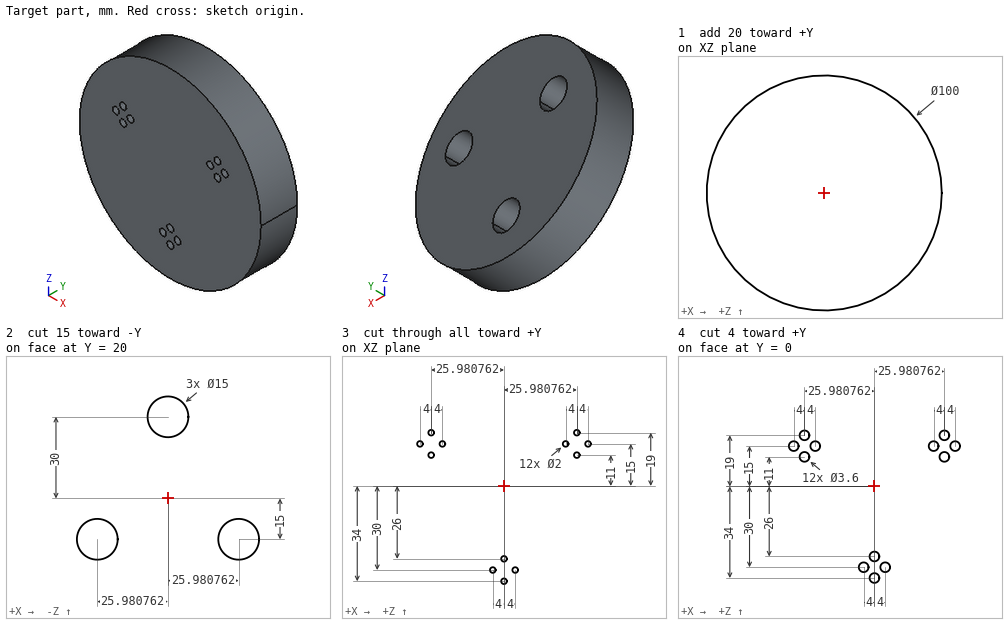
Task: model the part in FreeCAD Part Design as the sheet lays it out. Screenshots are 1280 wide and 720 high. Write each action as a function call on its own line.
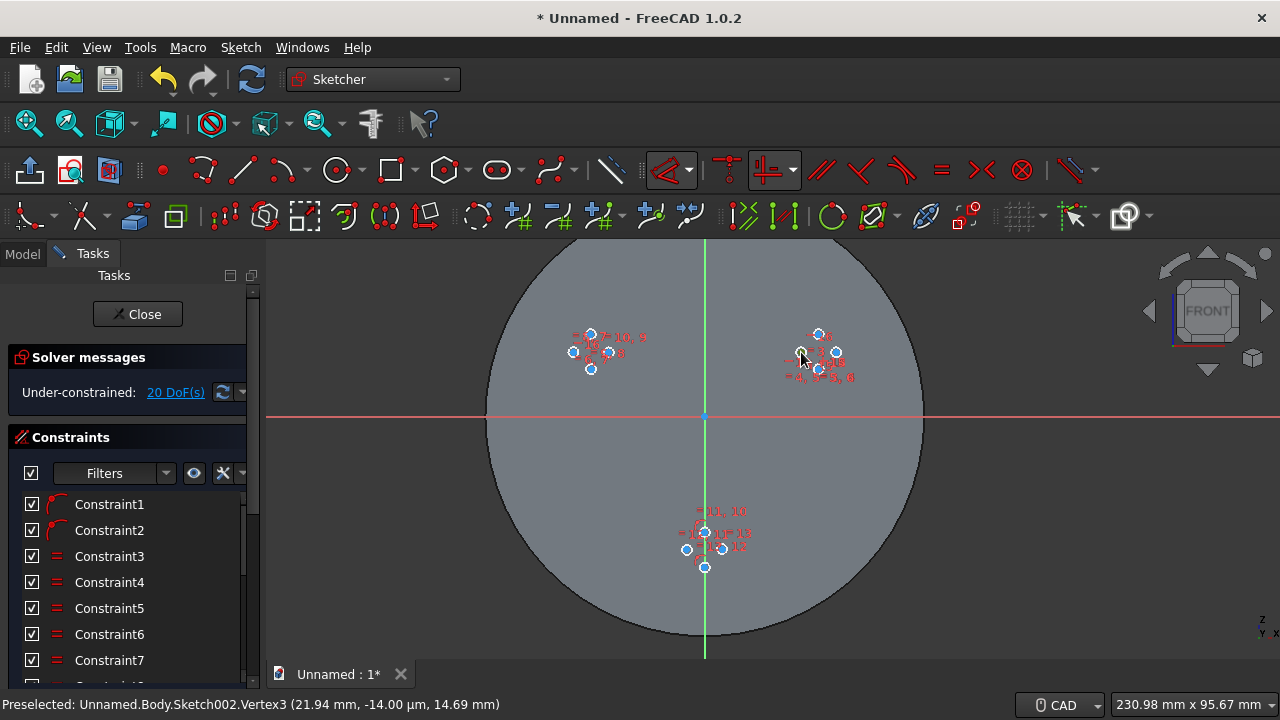
click(571, 354)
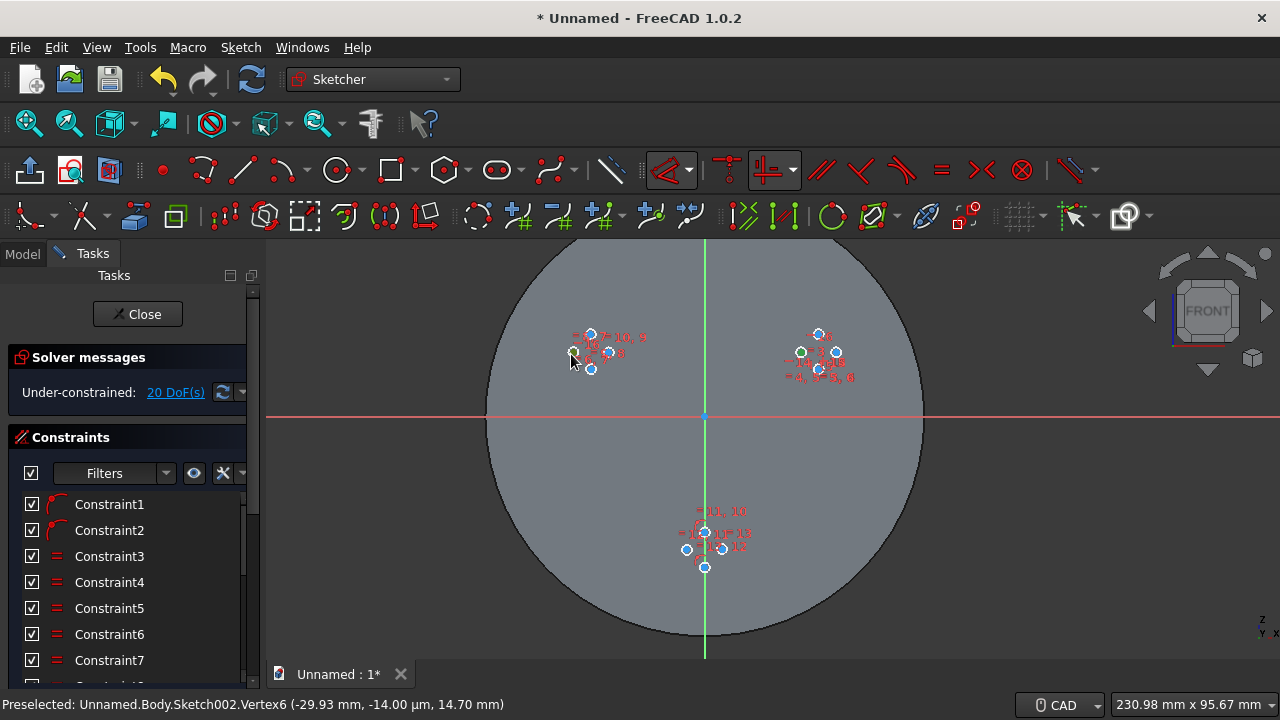
key(h)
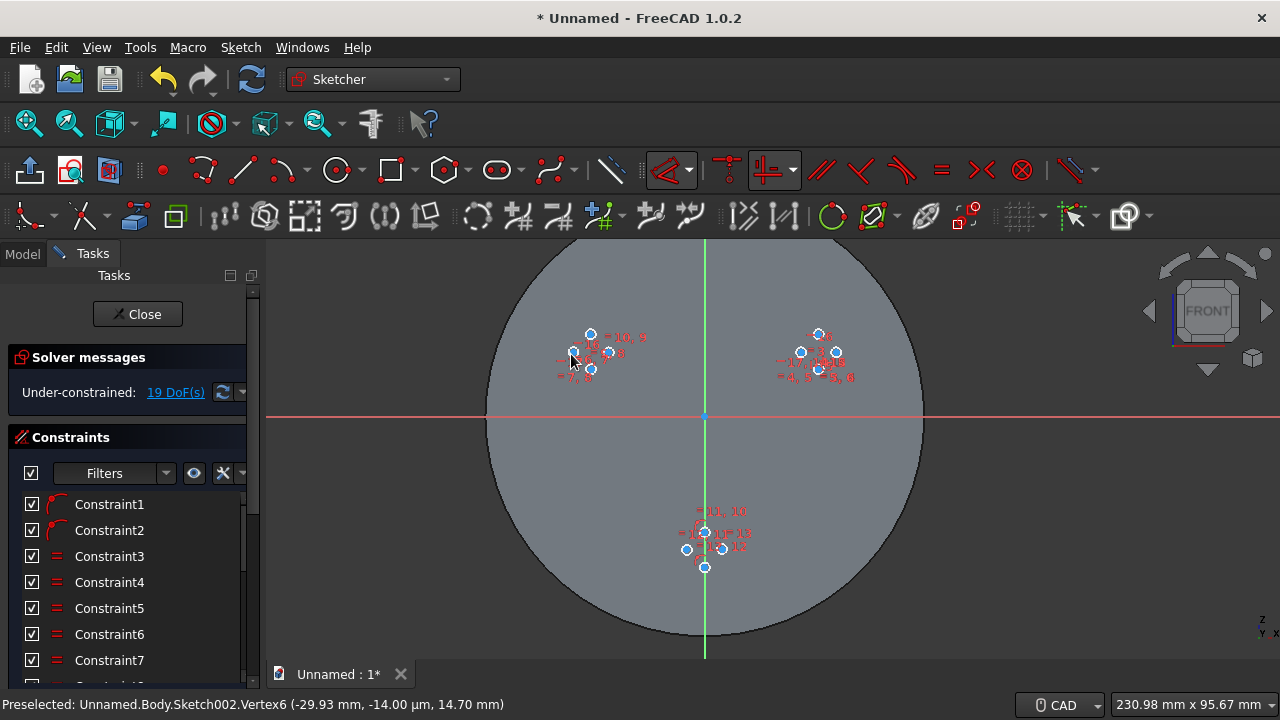
click(591, 334)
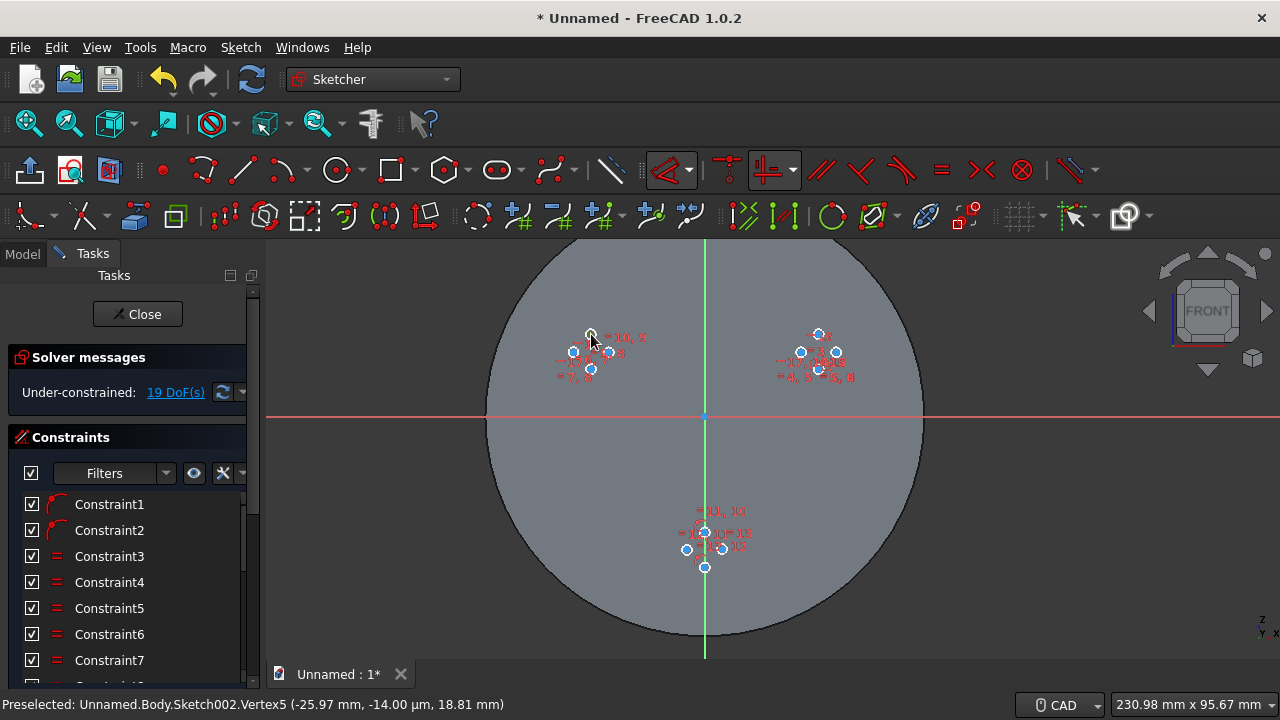
click(593, 371)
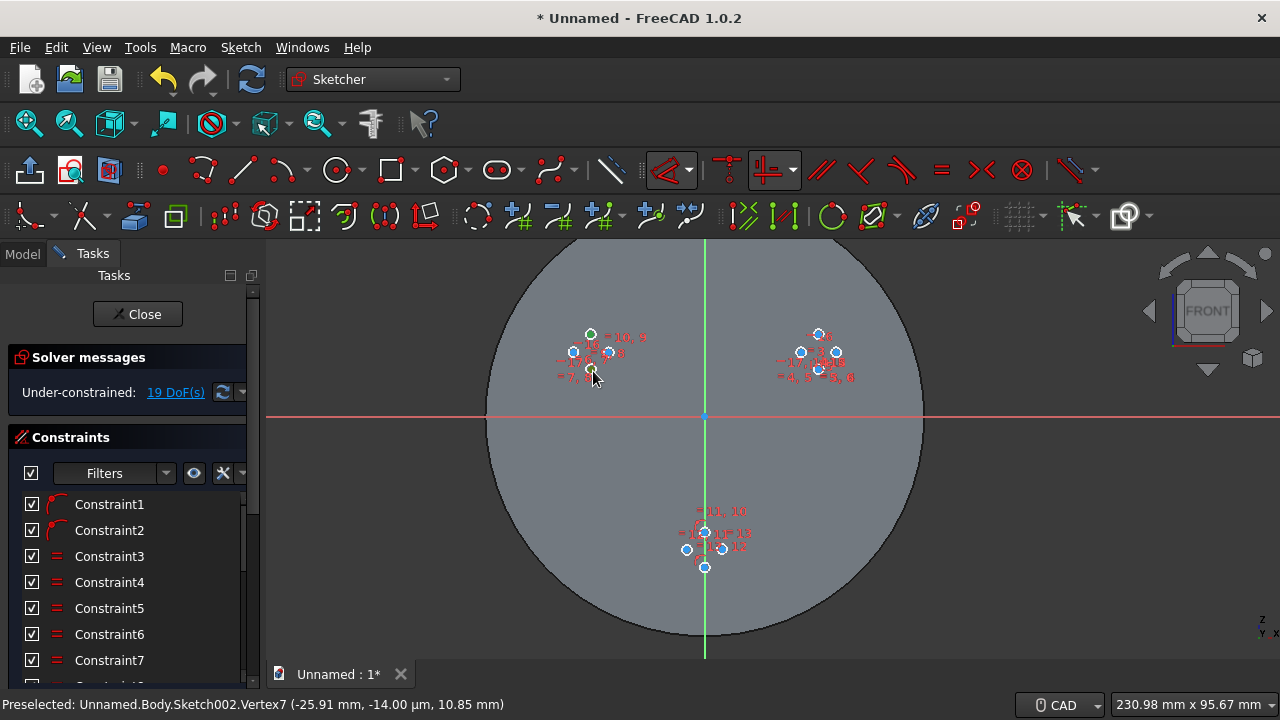
click(796, 170)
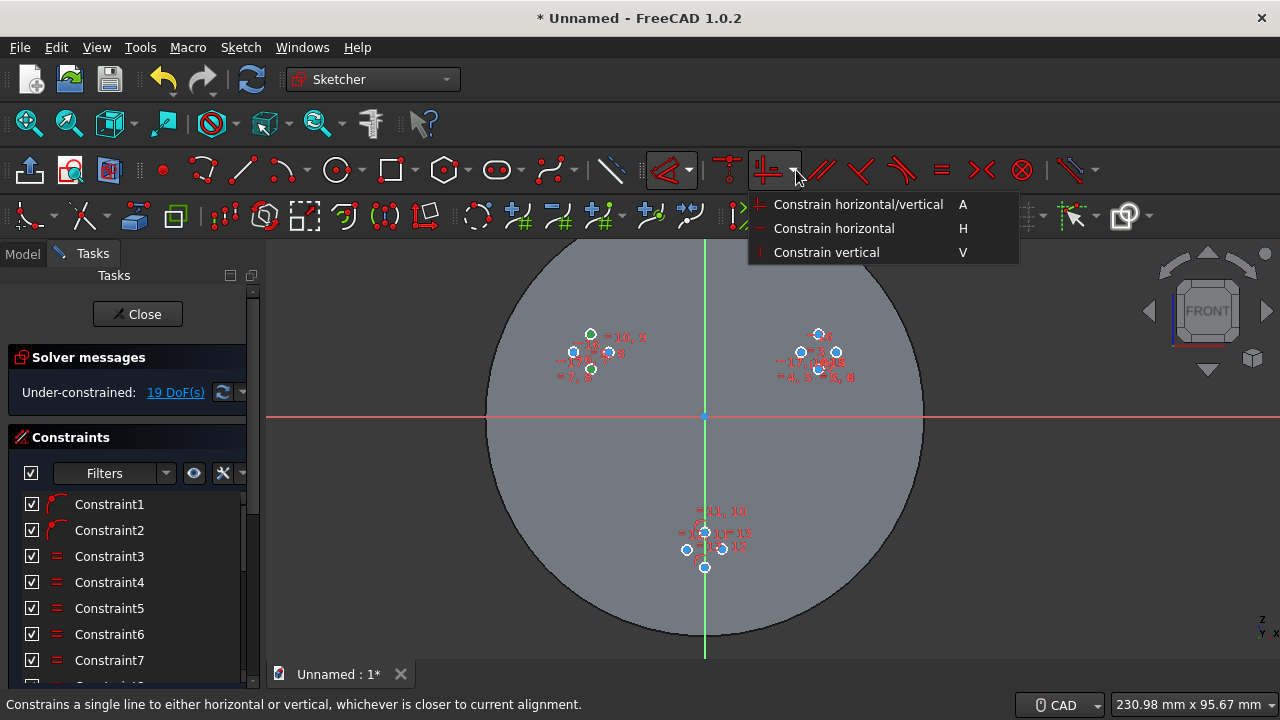
click(884, 252)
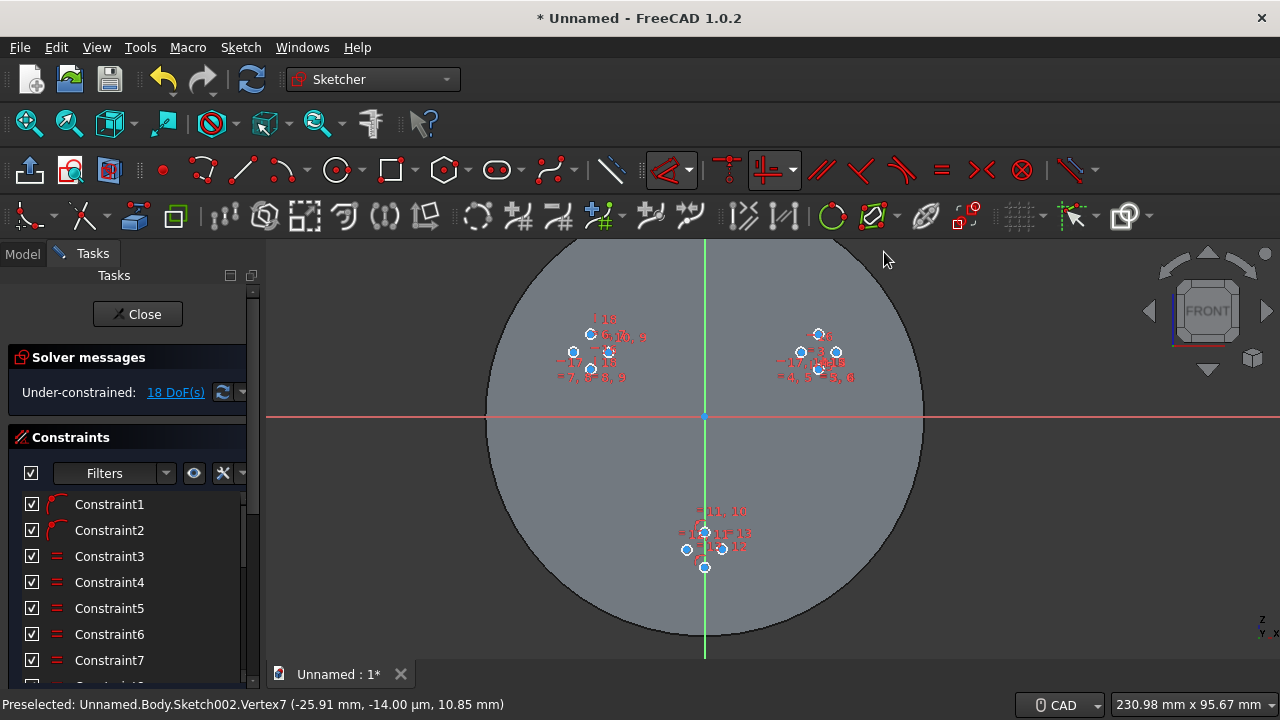
scroll(819, 369, up, 4)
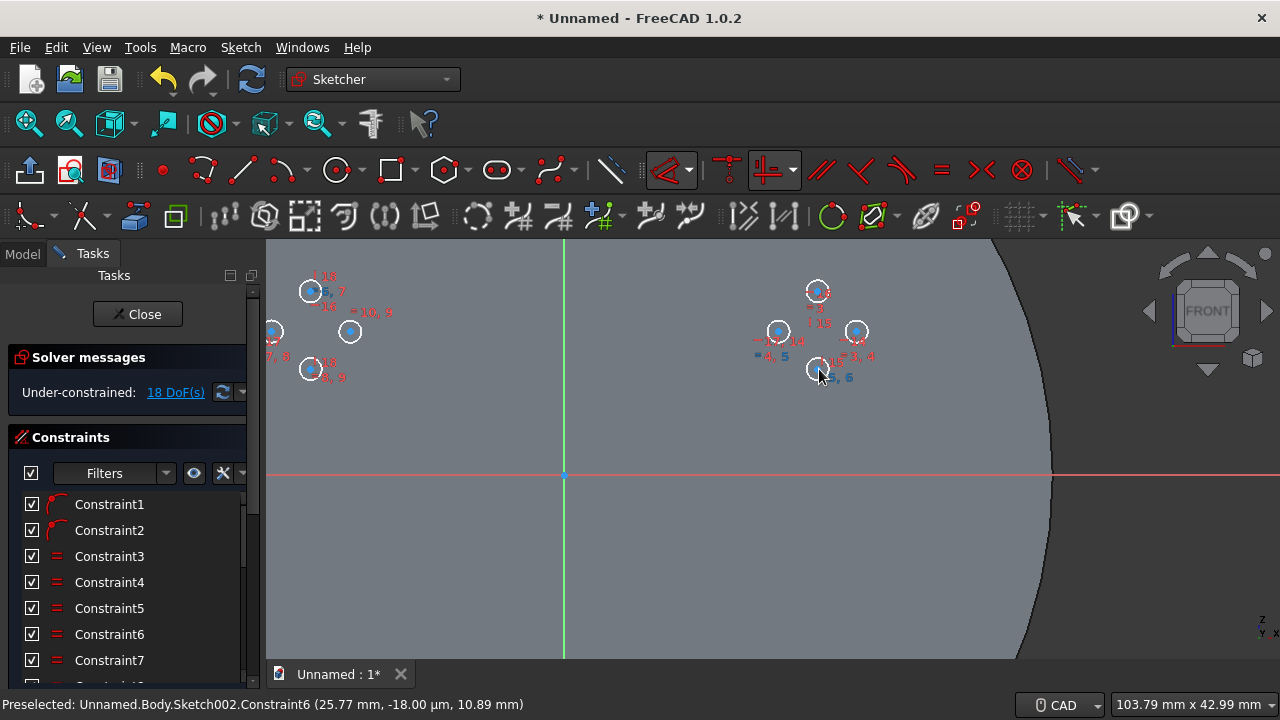
scroll(818, 369, up, 4)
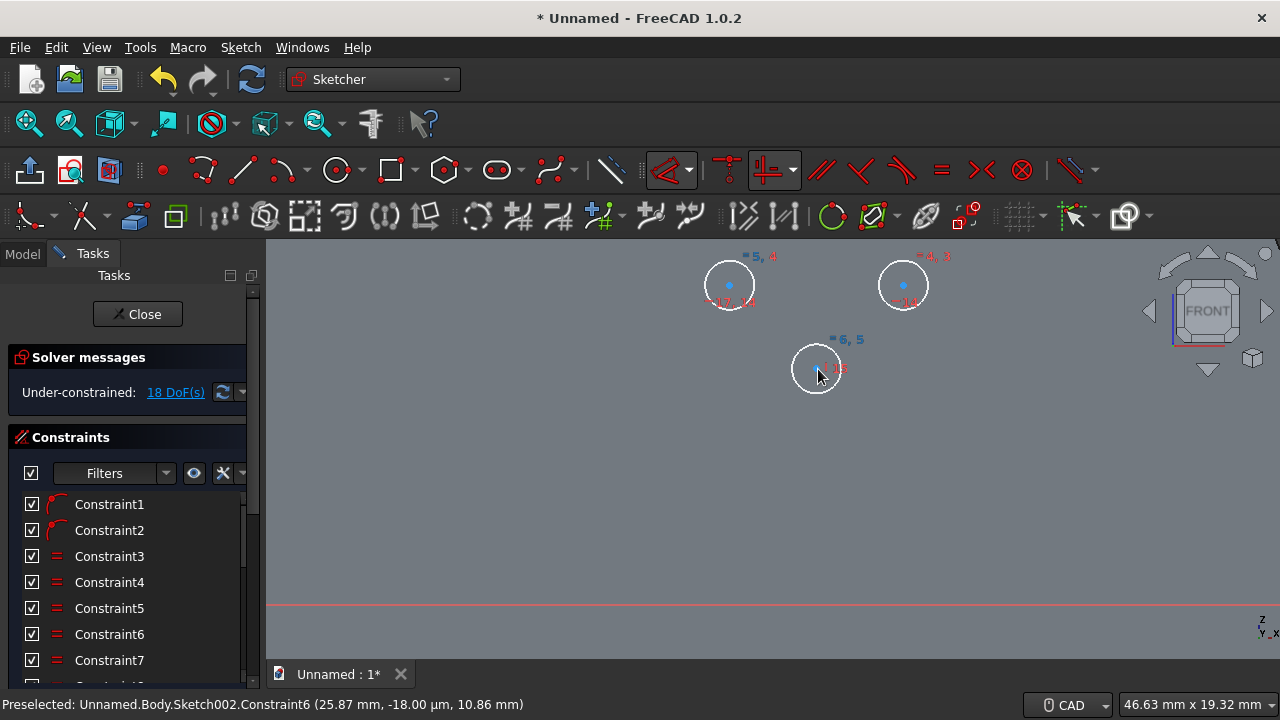
click(817, 369)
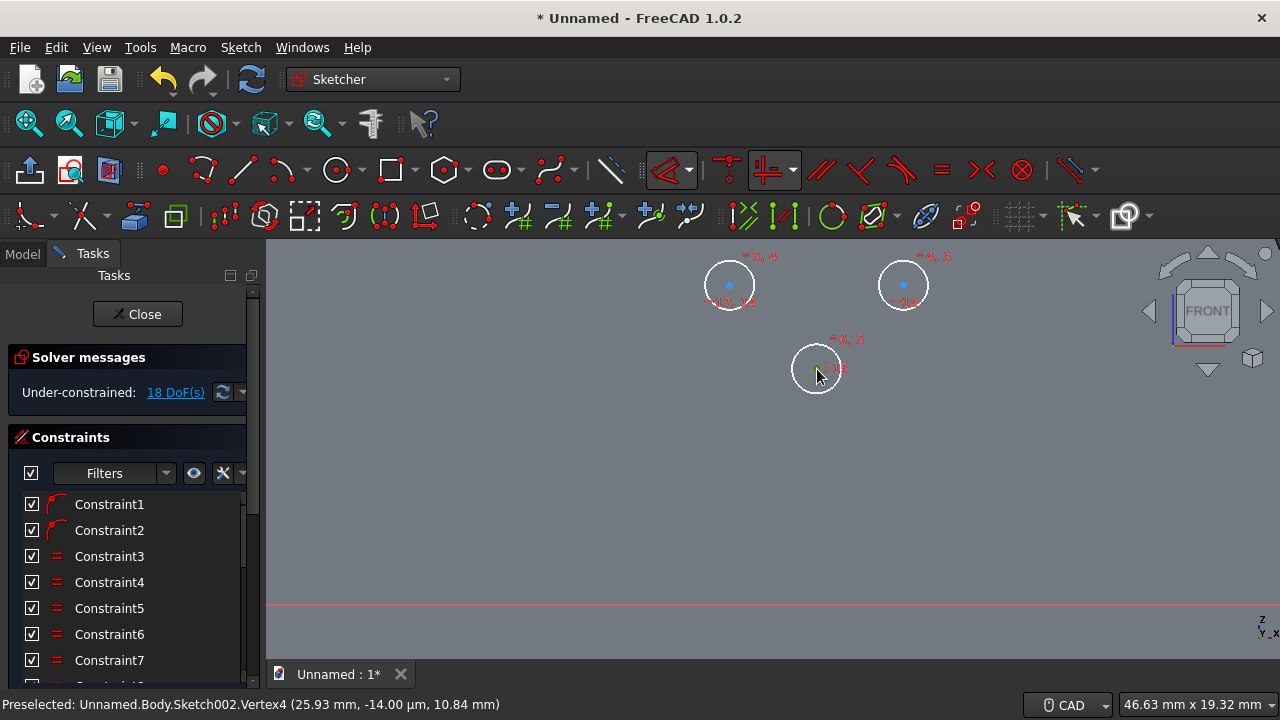
scroll(819, 368, down, 8)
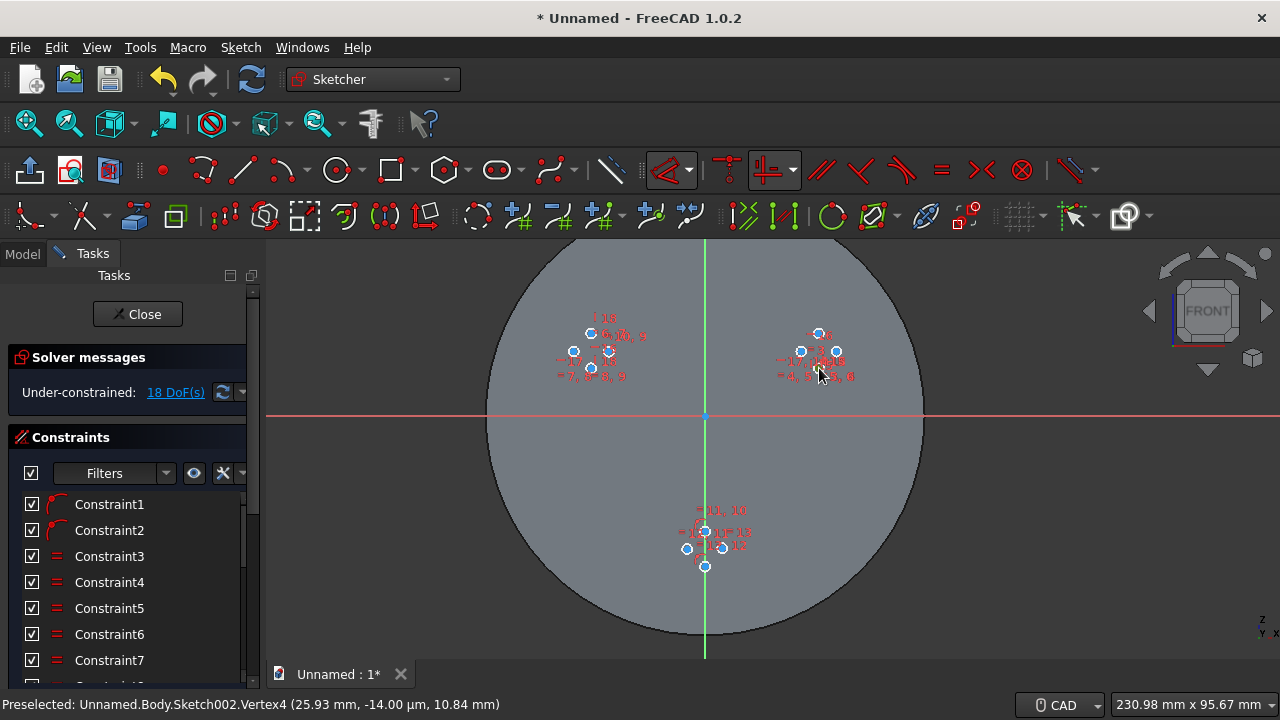
scroll(591, 368, up, 4)